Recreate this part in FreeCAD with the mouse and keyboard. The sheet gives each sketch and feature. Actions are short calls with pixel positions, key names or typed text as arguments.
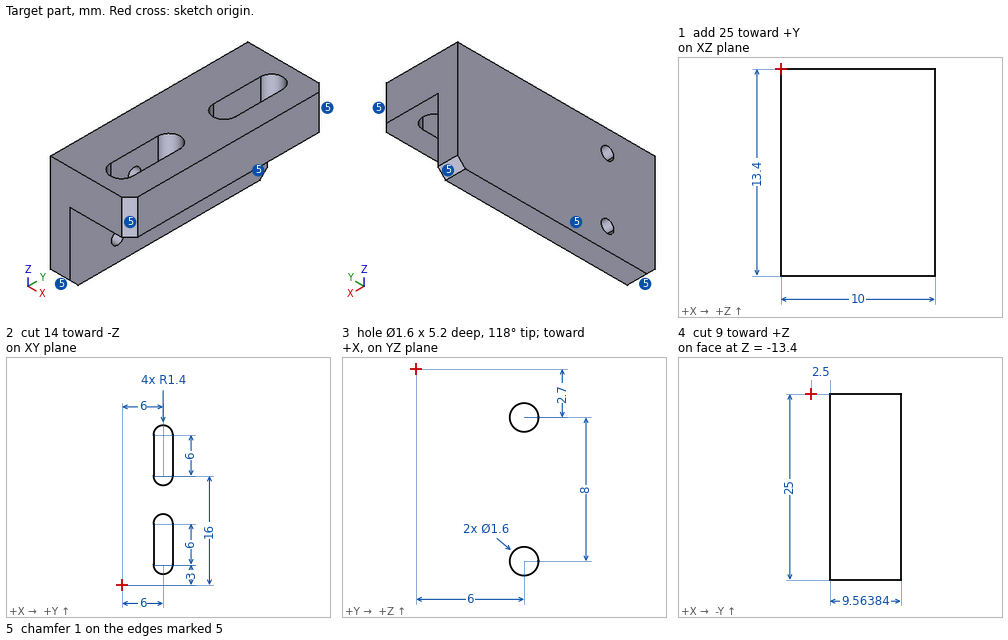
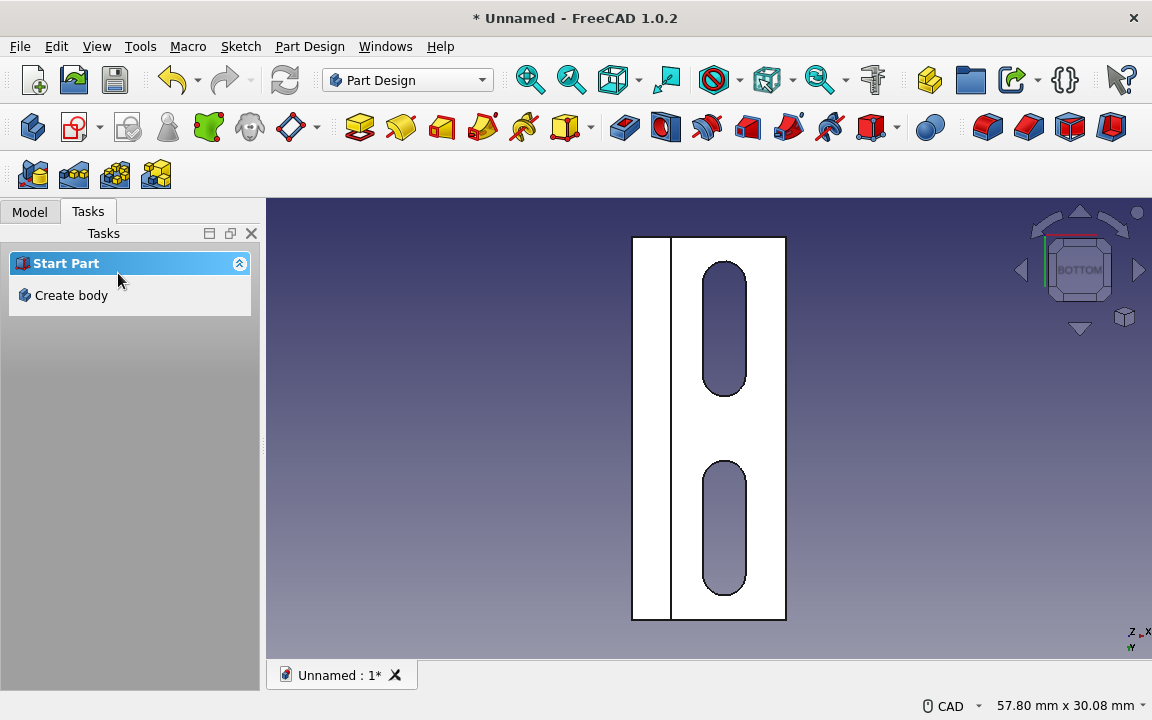
click(652, 236)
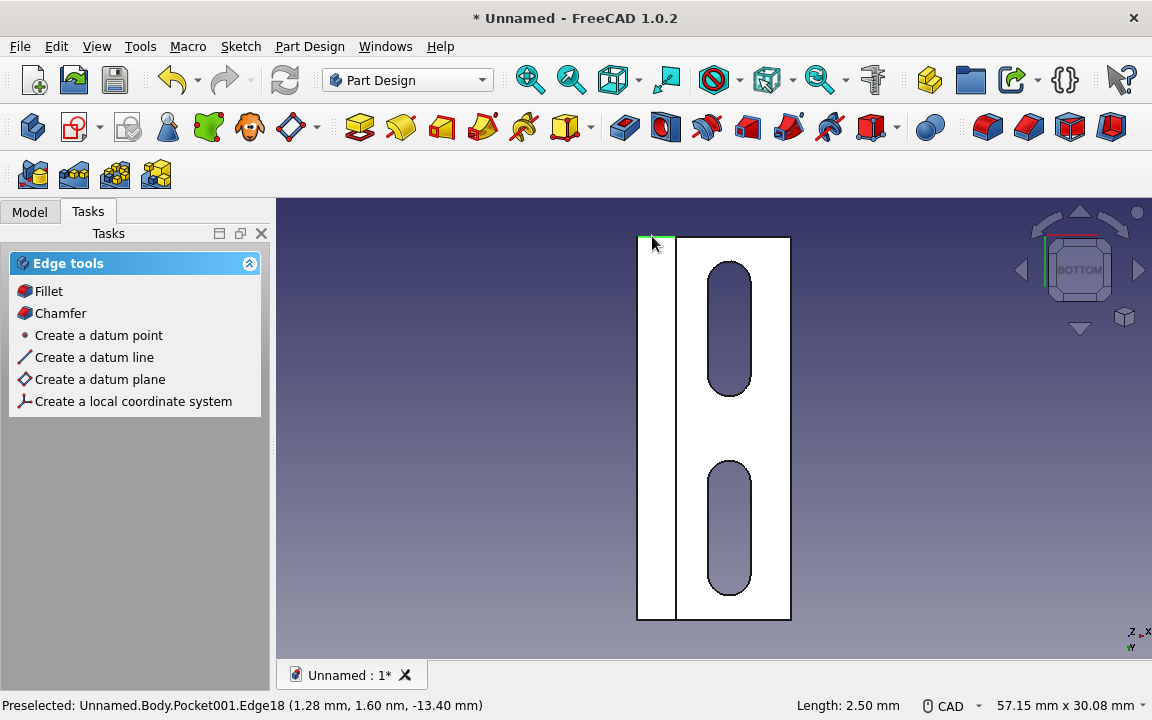
key(0)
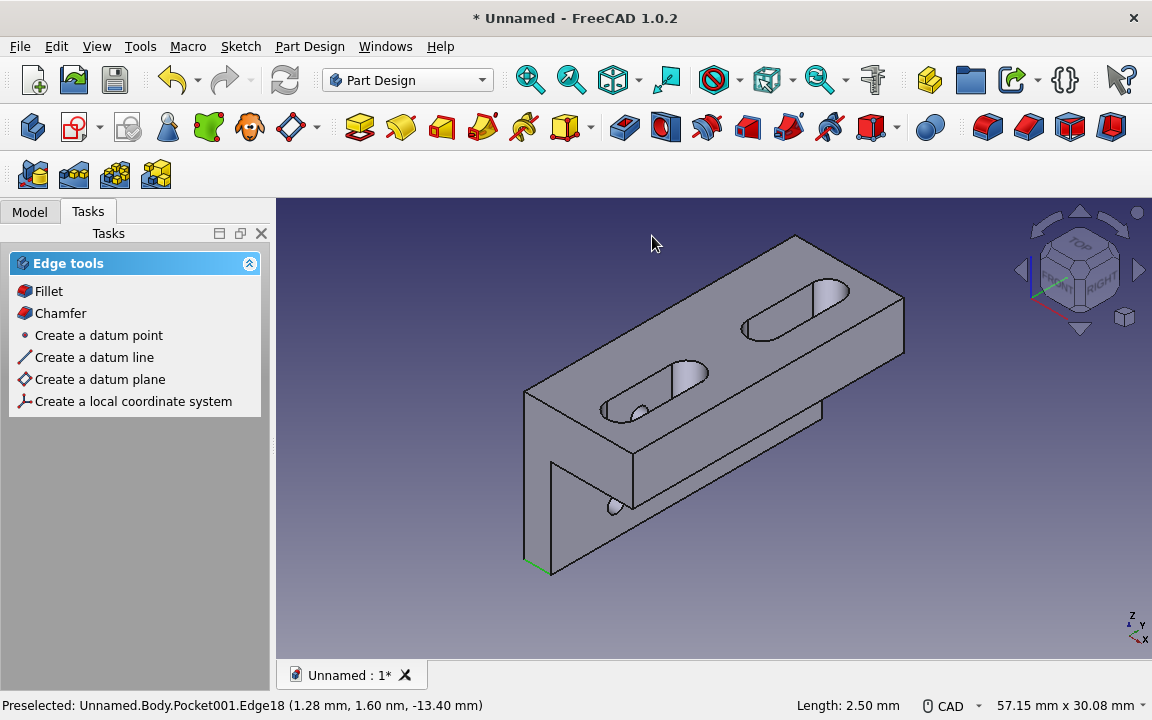
click(633, 481, ctrl)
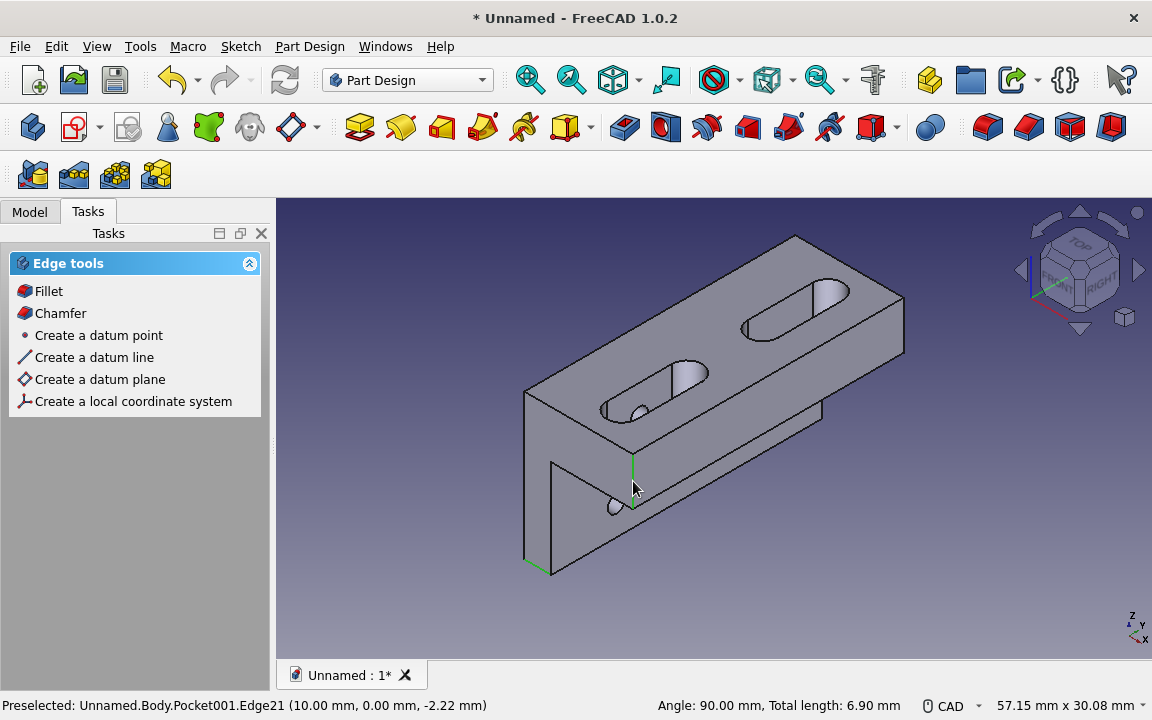
key(2)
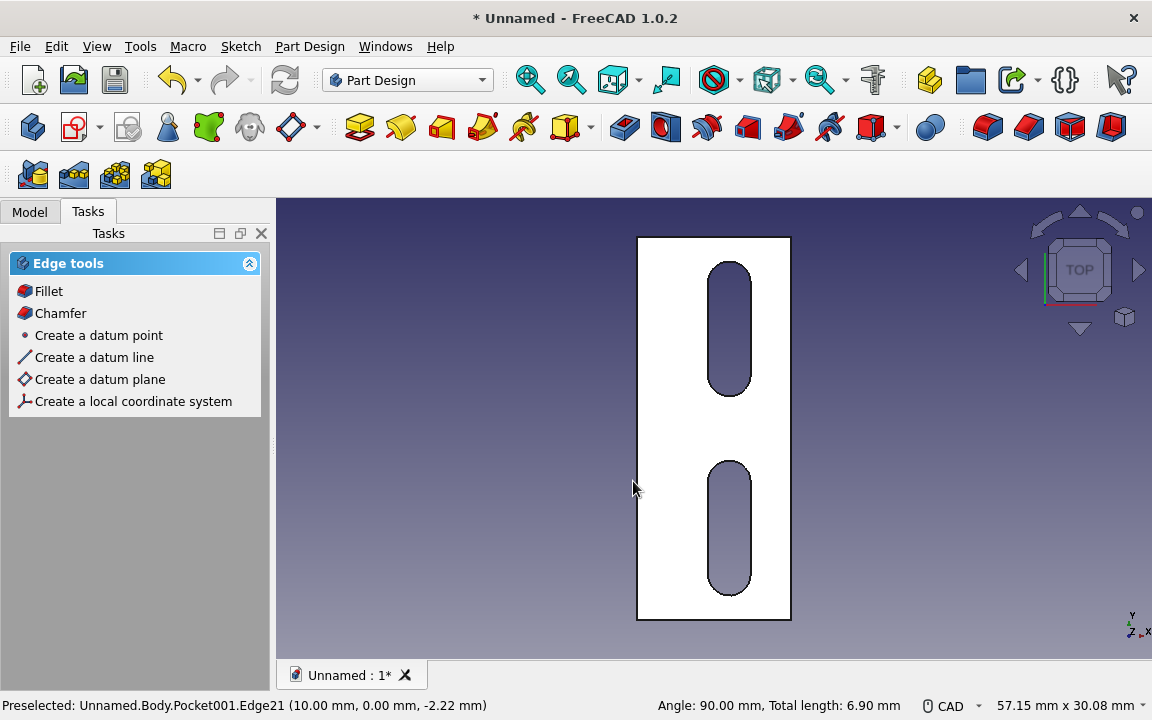
key(1)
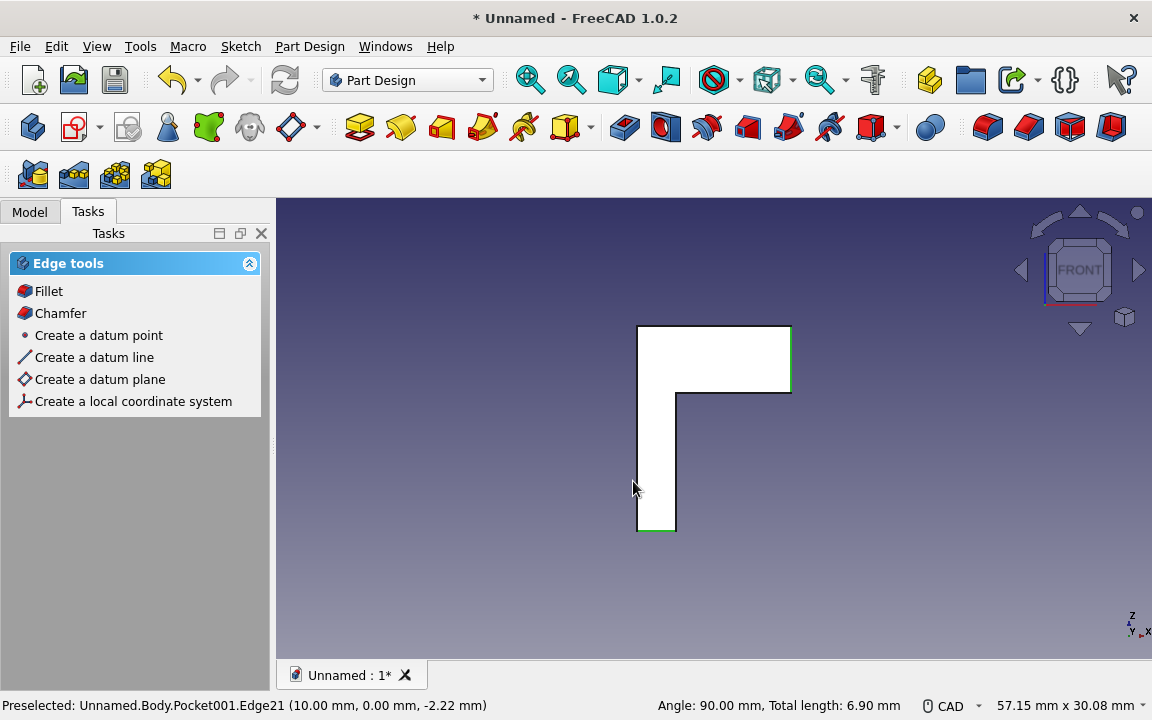
key(v)
key(f)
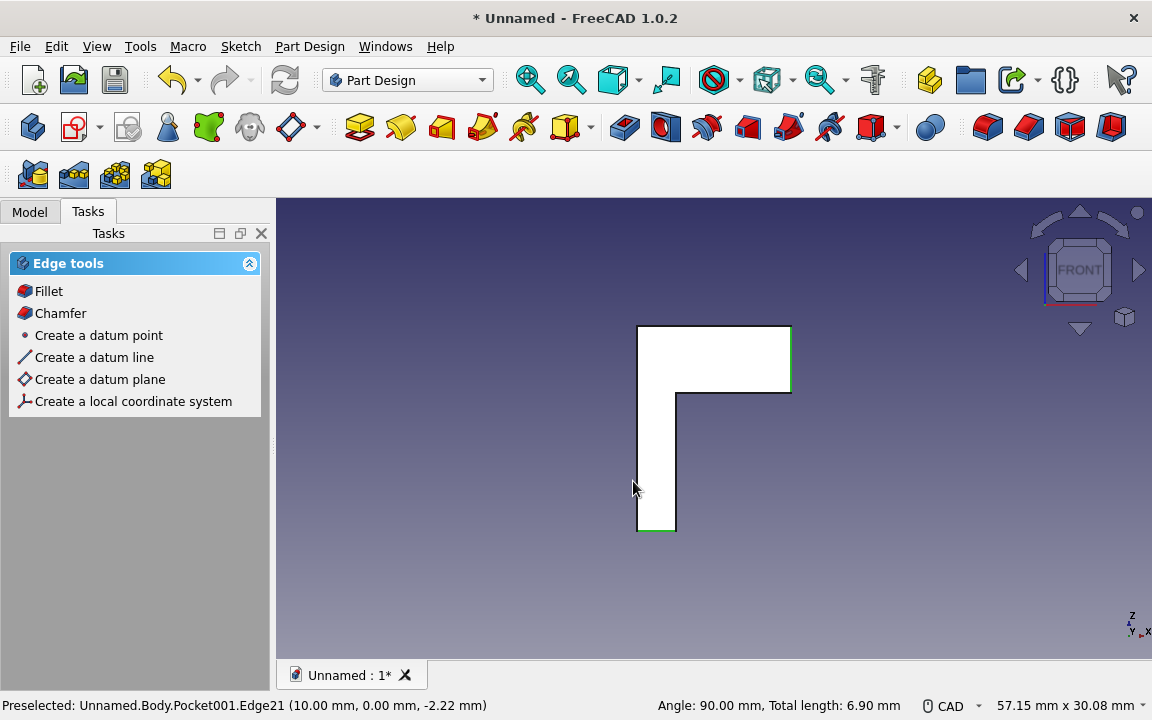
key(3)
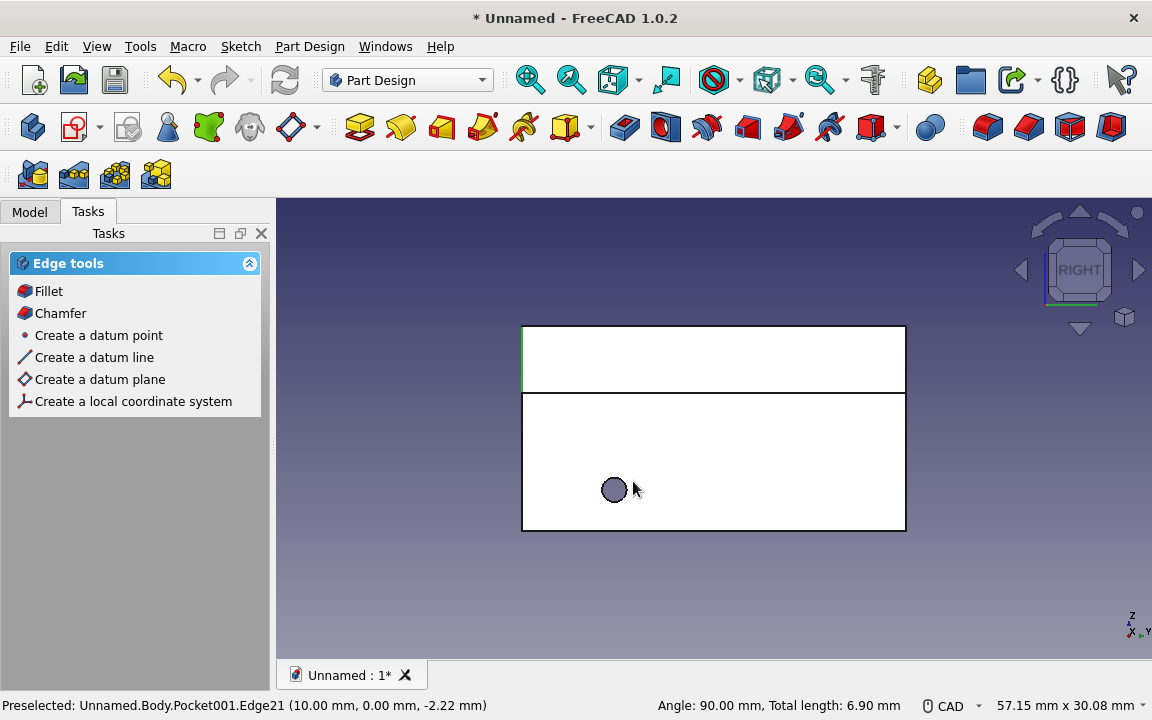
click(531, 80)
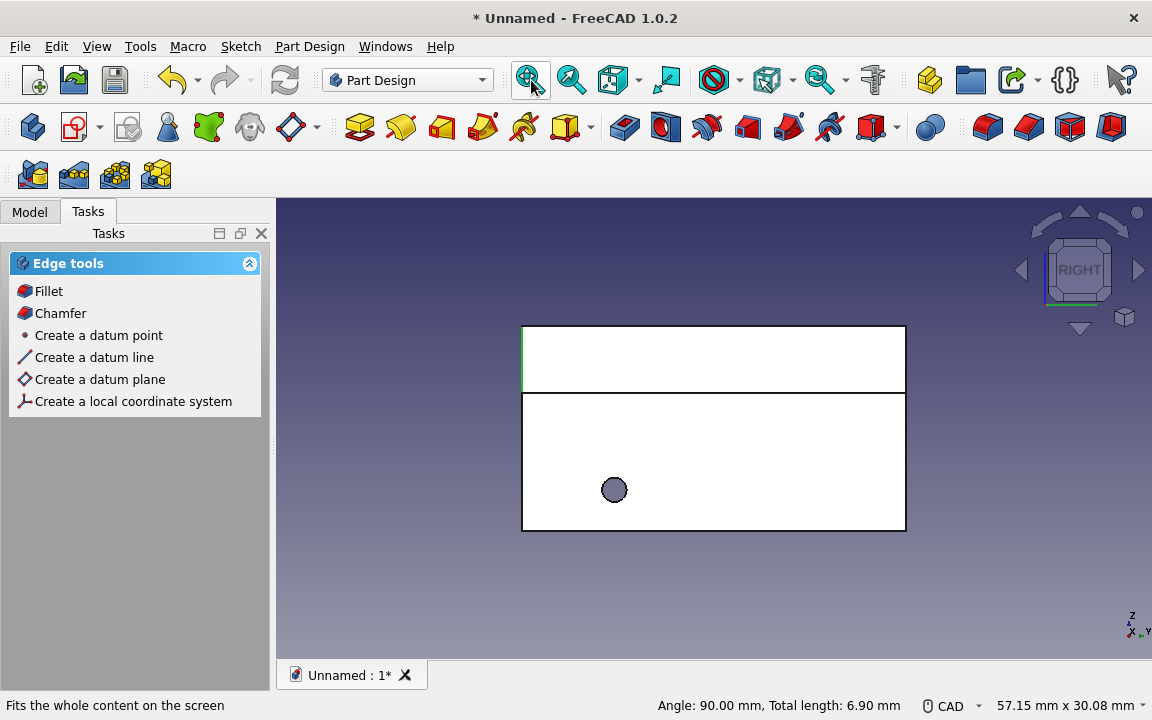
click(906, 359, ctrl)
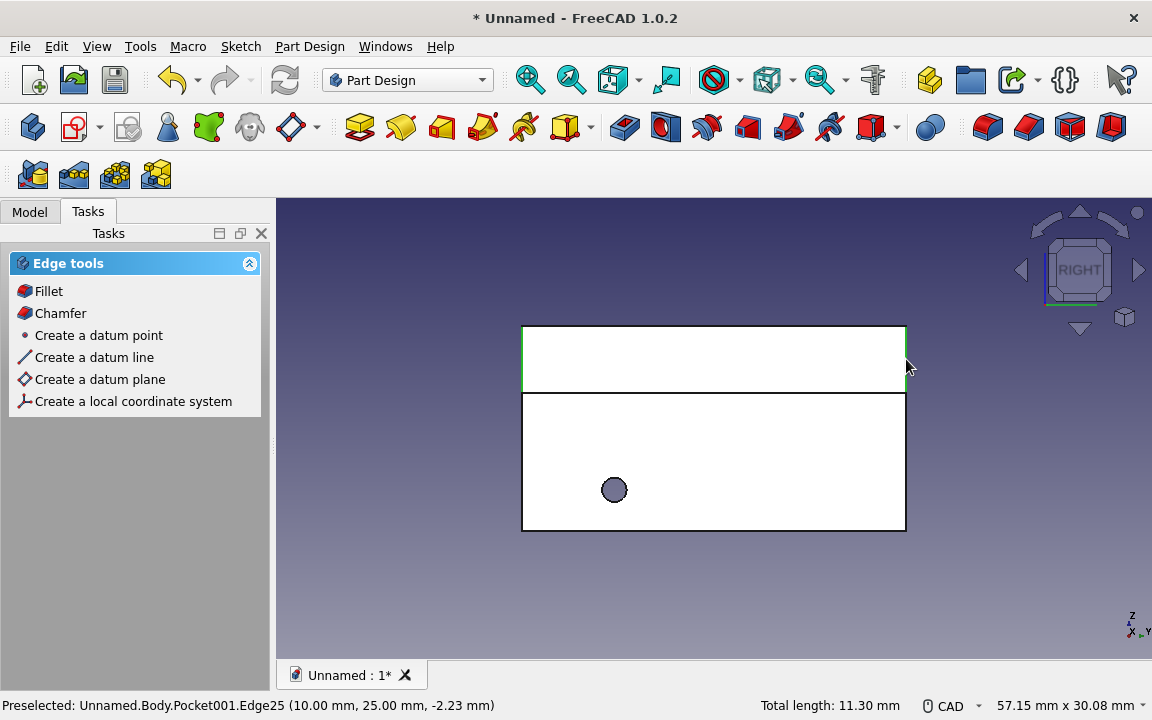
key(5)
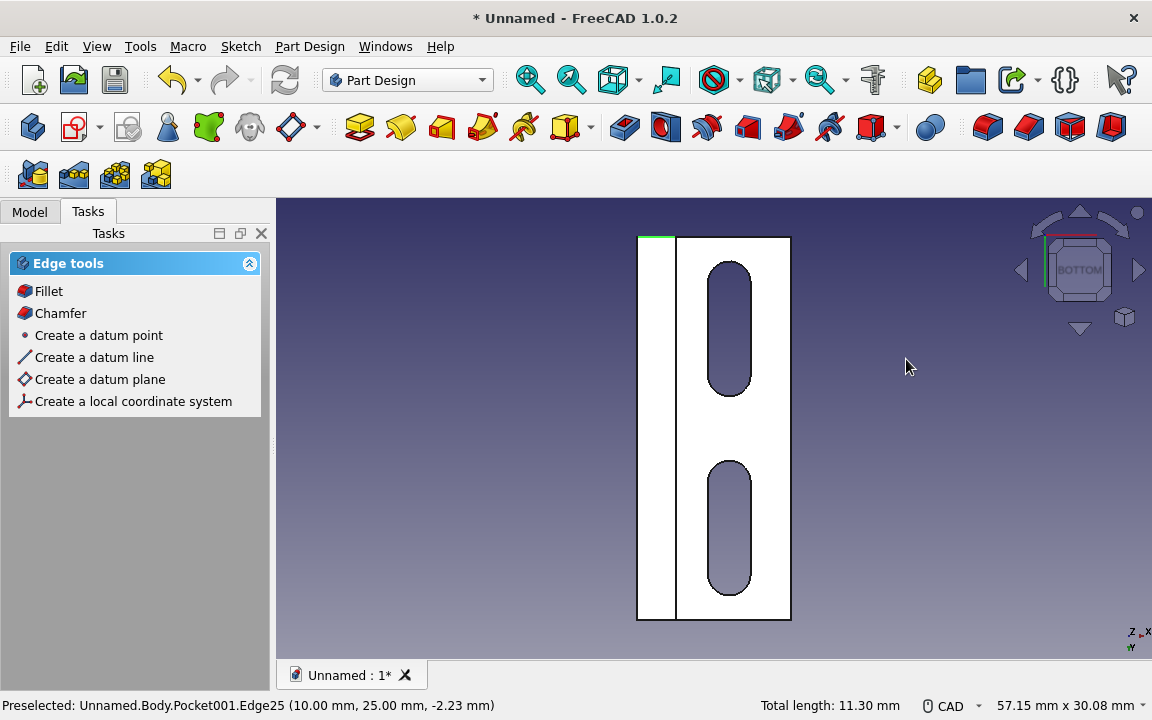
key(4)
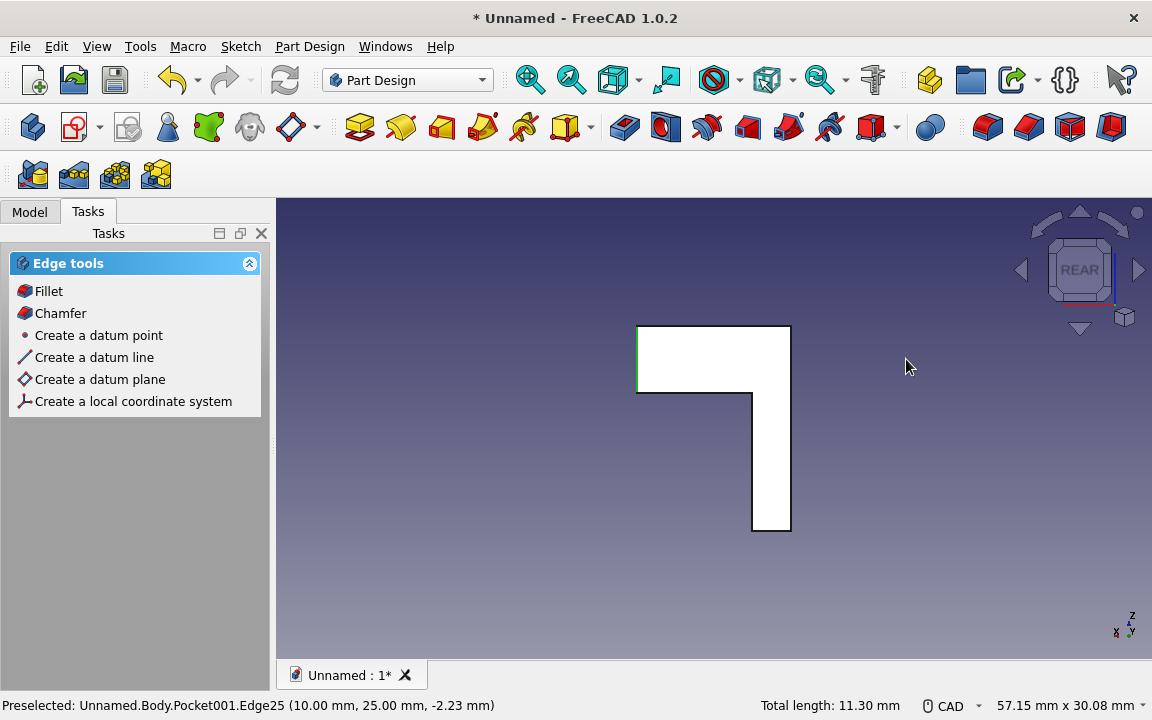
click(531, 80)